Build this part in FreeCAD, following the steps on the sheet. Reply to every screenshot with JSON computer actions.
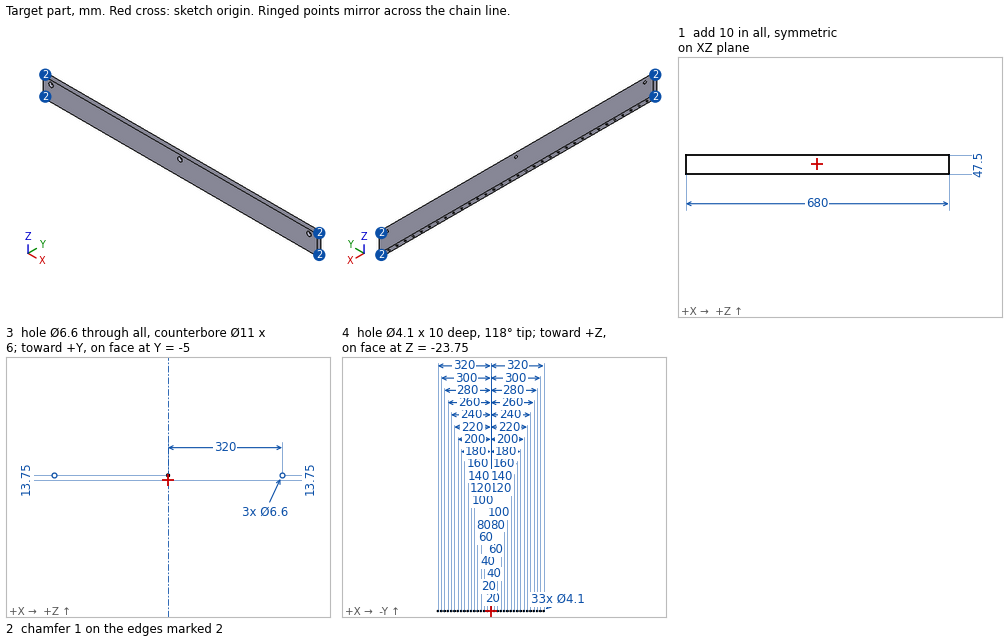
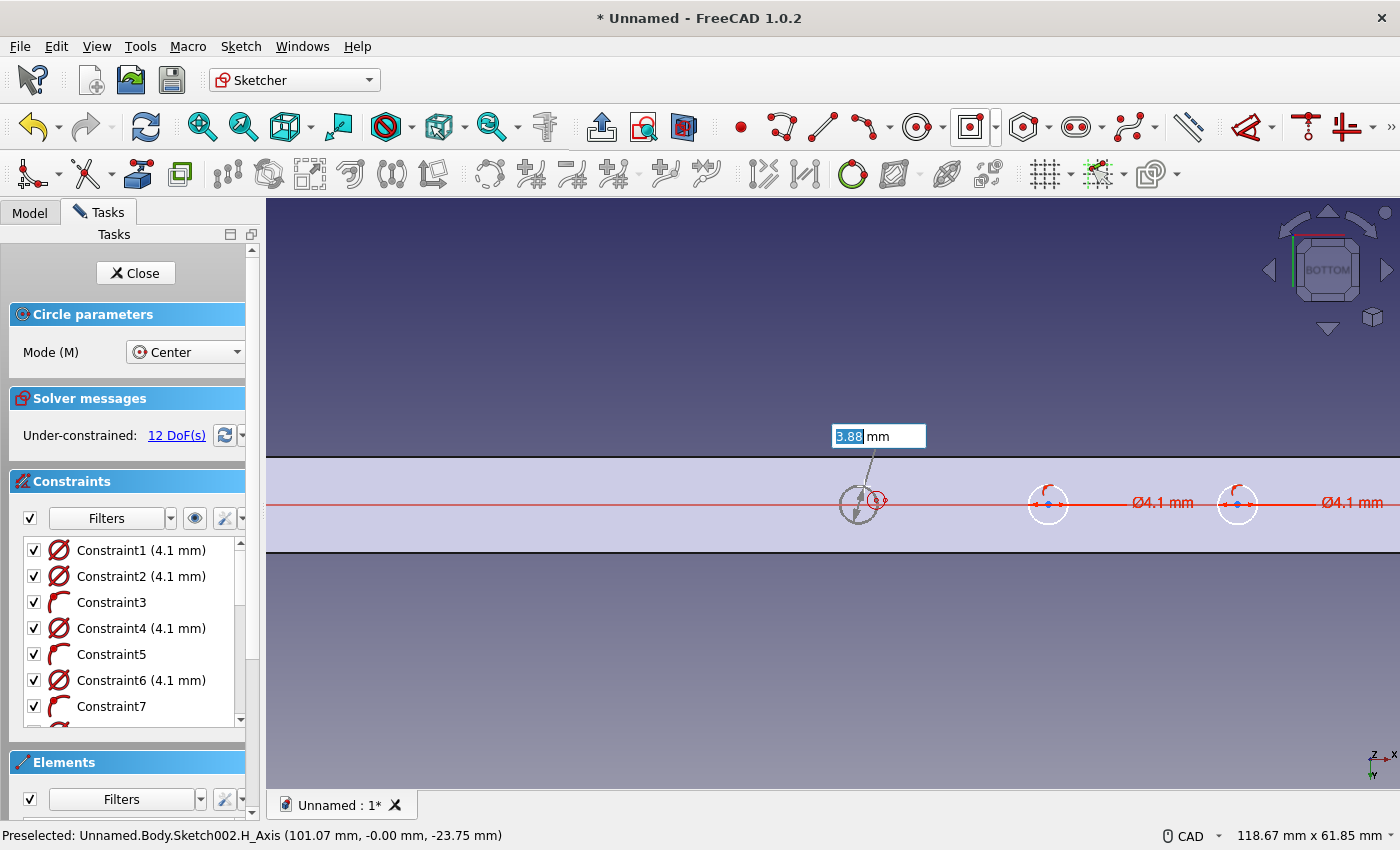
{"action": "type", "text": "4.1"}
{"action": "key", "text": "Return"}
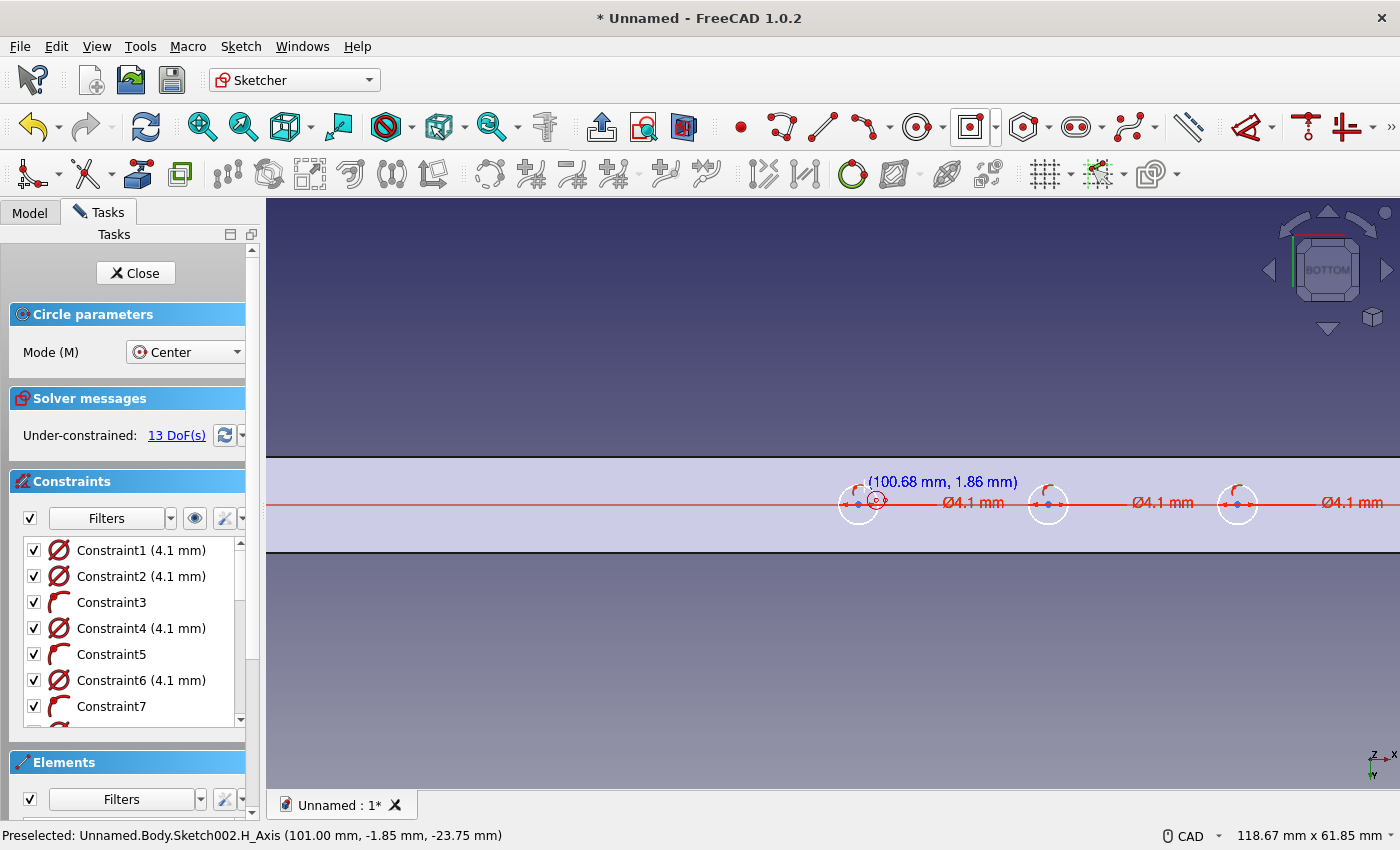
{"action": "scroll", "coordinate": [872, 492], "scroll_direction": "down", "scroll_amount": 11}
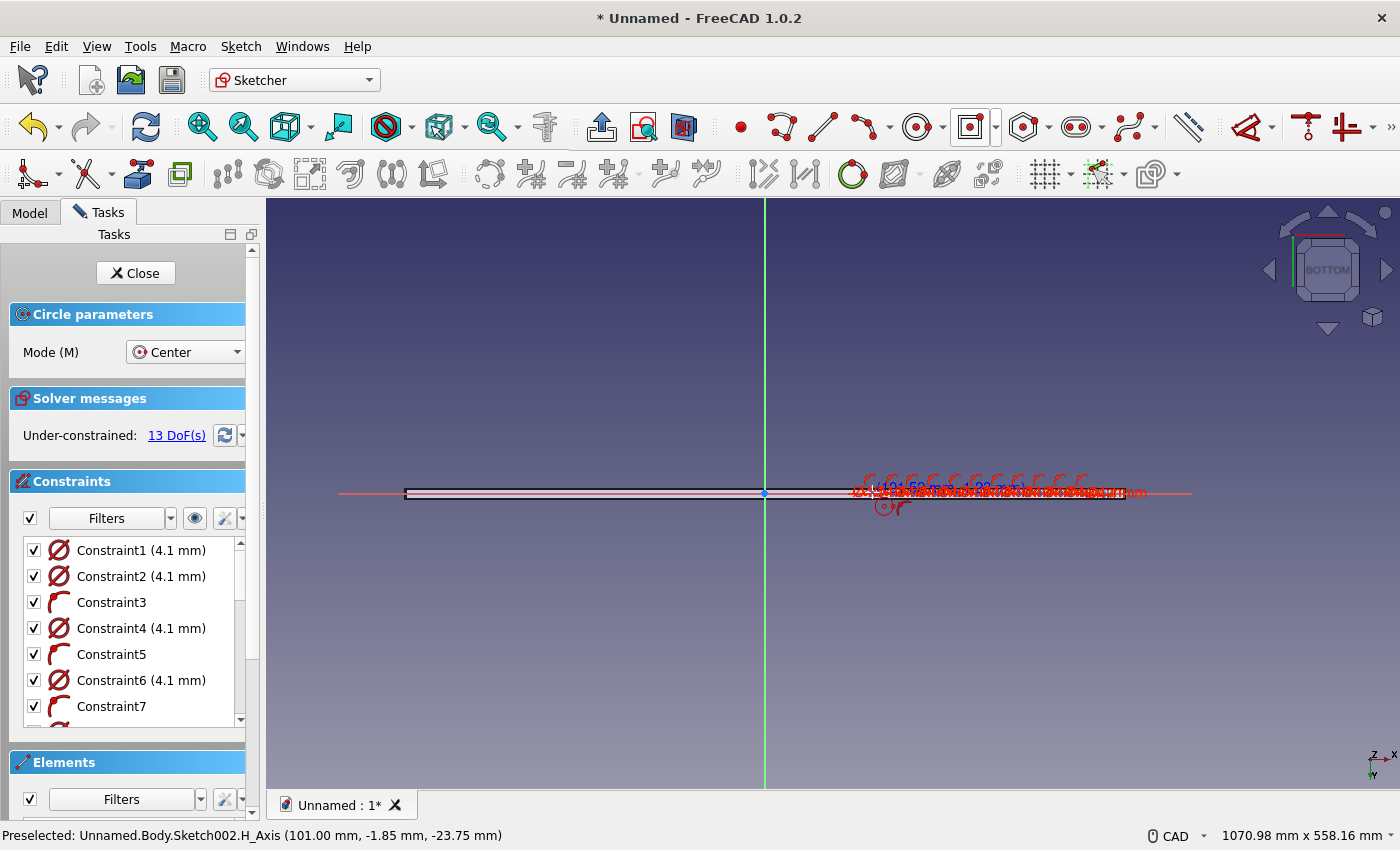
{"action": "left_click", "coordinate": [850, 494]}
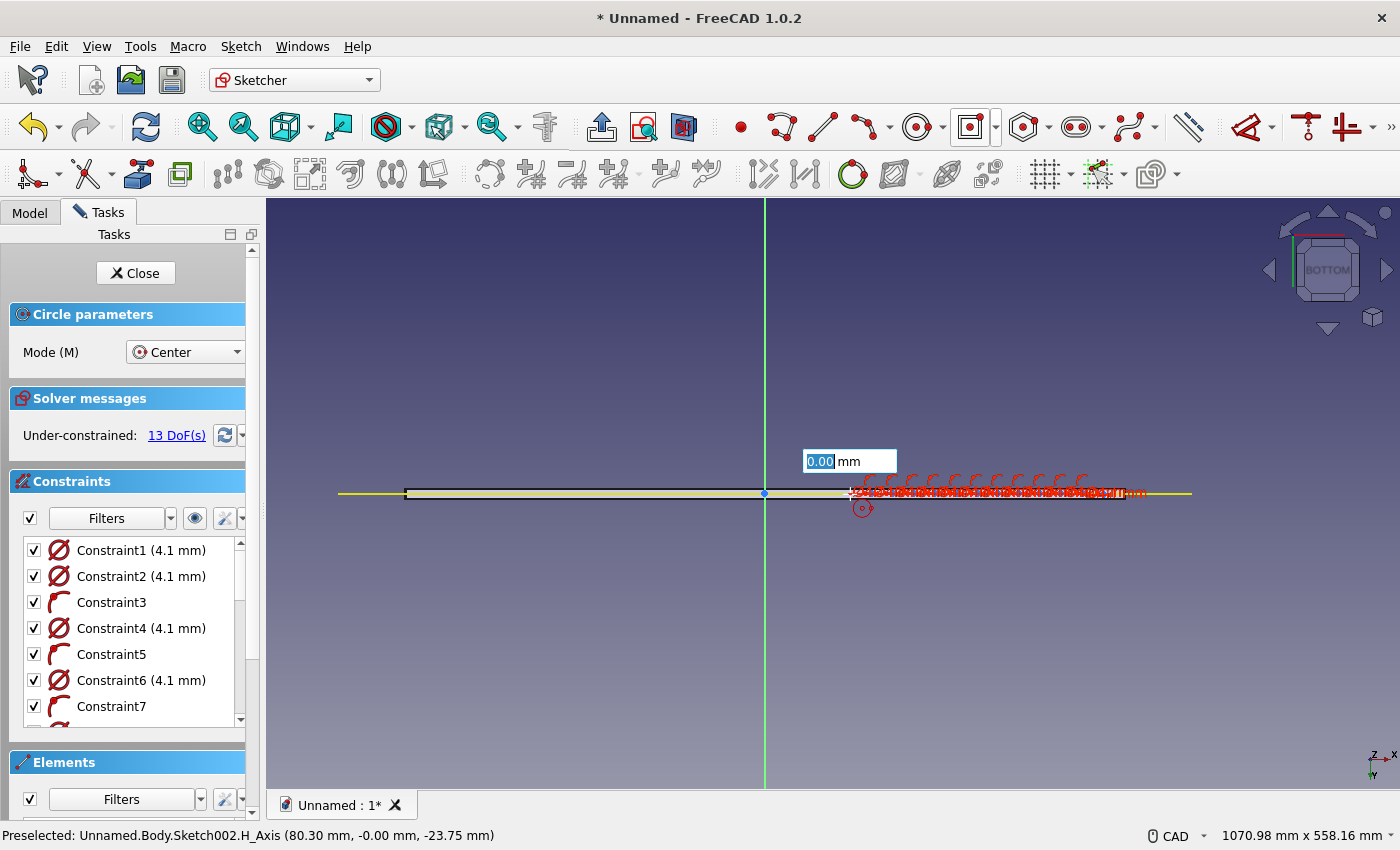
{"action": "scroll", "coordinate": [849, 496], "scroll_direction": "up", "scroll_amount": 11}
{"action": "mouse_move", "coordinate": [844, 491]}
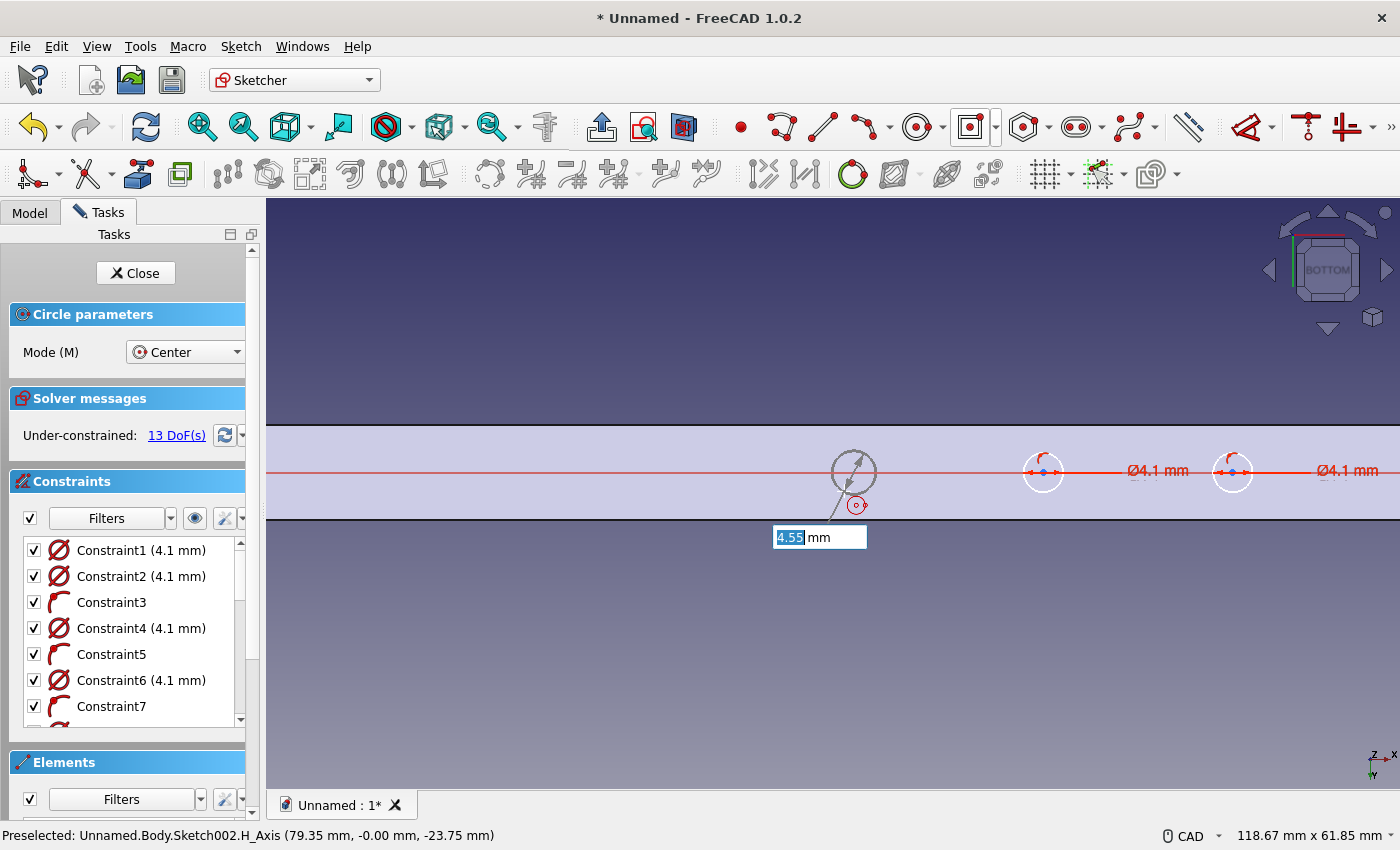
{"action": "type", "text": "4.1"}
{"action": "key", "text": "Return"}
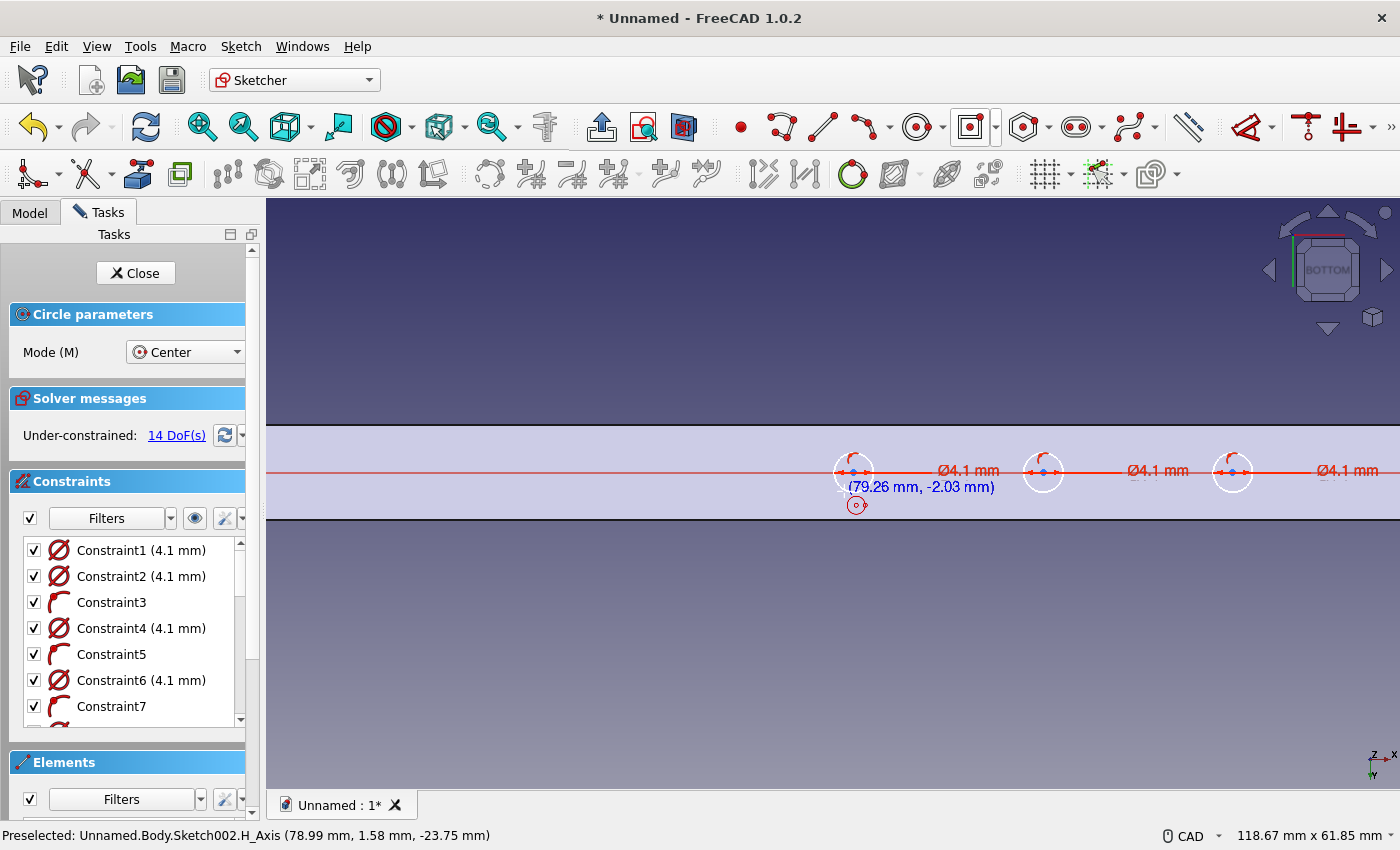
{"action": "scroll", "coordinate": [849, 496], "scroll_direction": "down", "scroll_amount": 11}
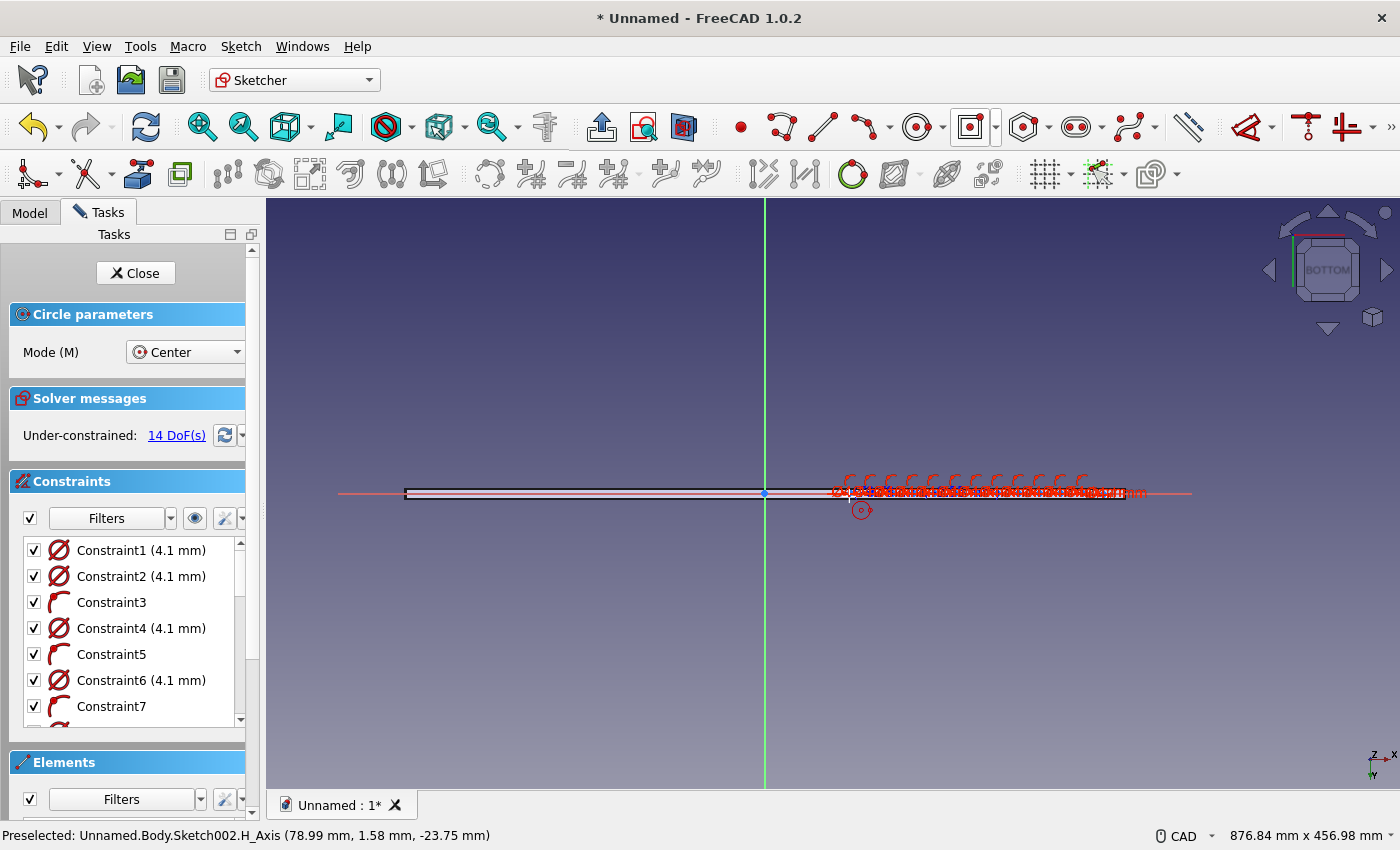
{"action": "left_click", "coordinate": [829, 494]}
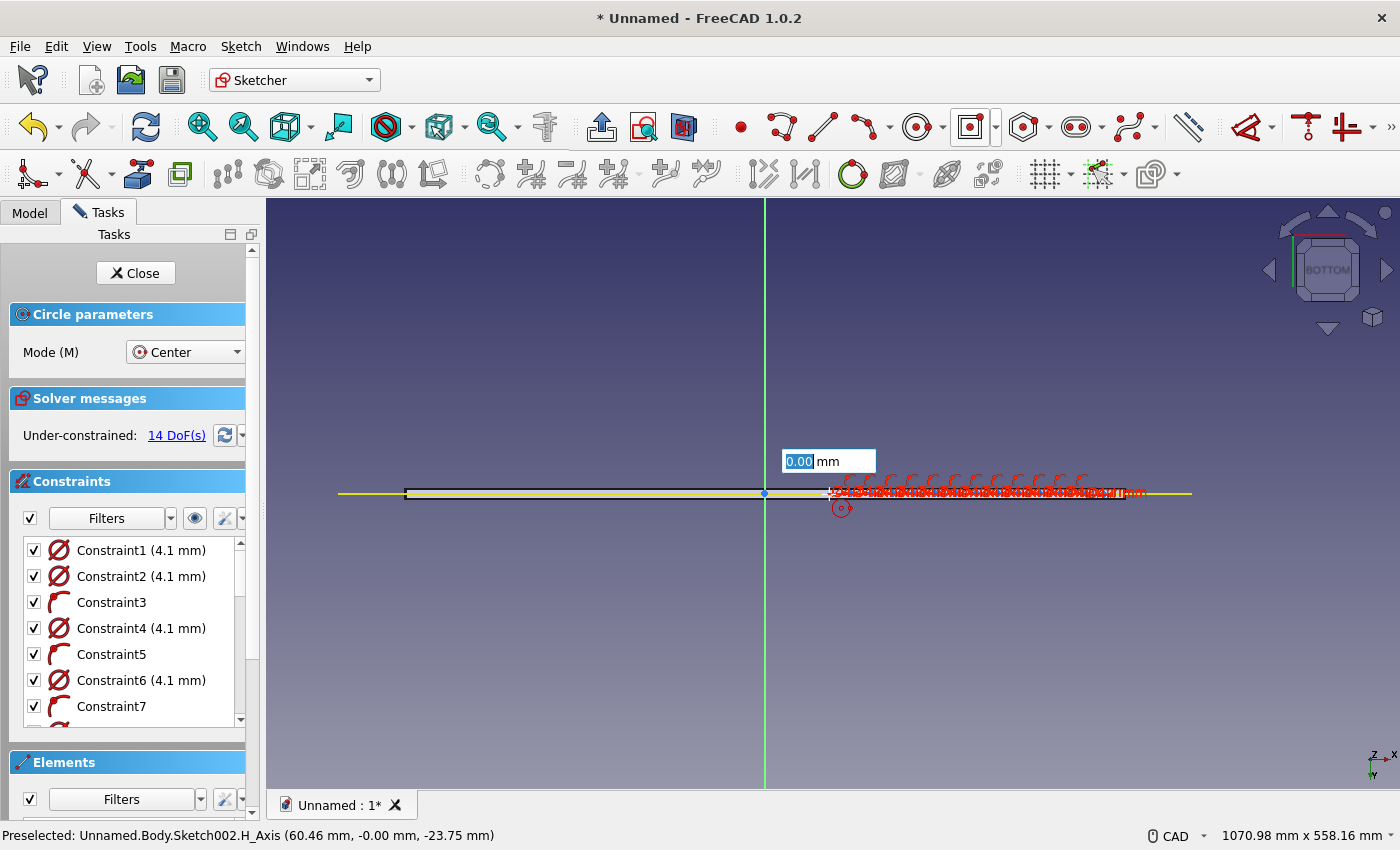
{"action": "scroll", "coordinate": [828, 496], "scroll_direction": "up", "scroll_amount": 11}
{"action": "mouse_move", "coordinate": [822, 491]}